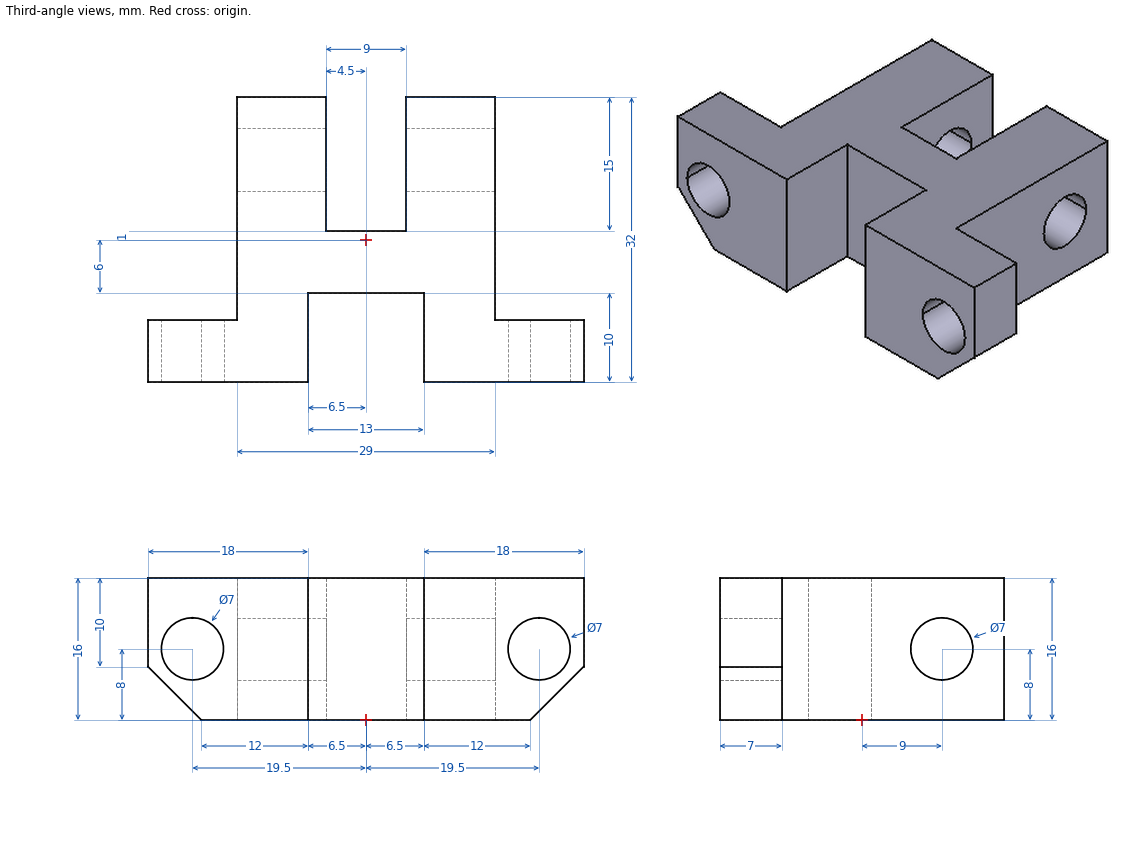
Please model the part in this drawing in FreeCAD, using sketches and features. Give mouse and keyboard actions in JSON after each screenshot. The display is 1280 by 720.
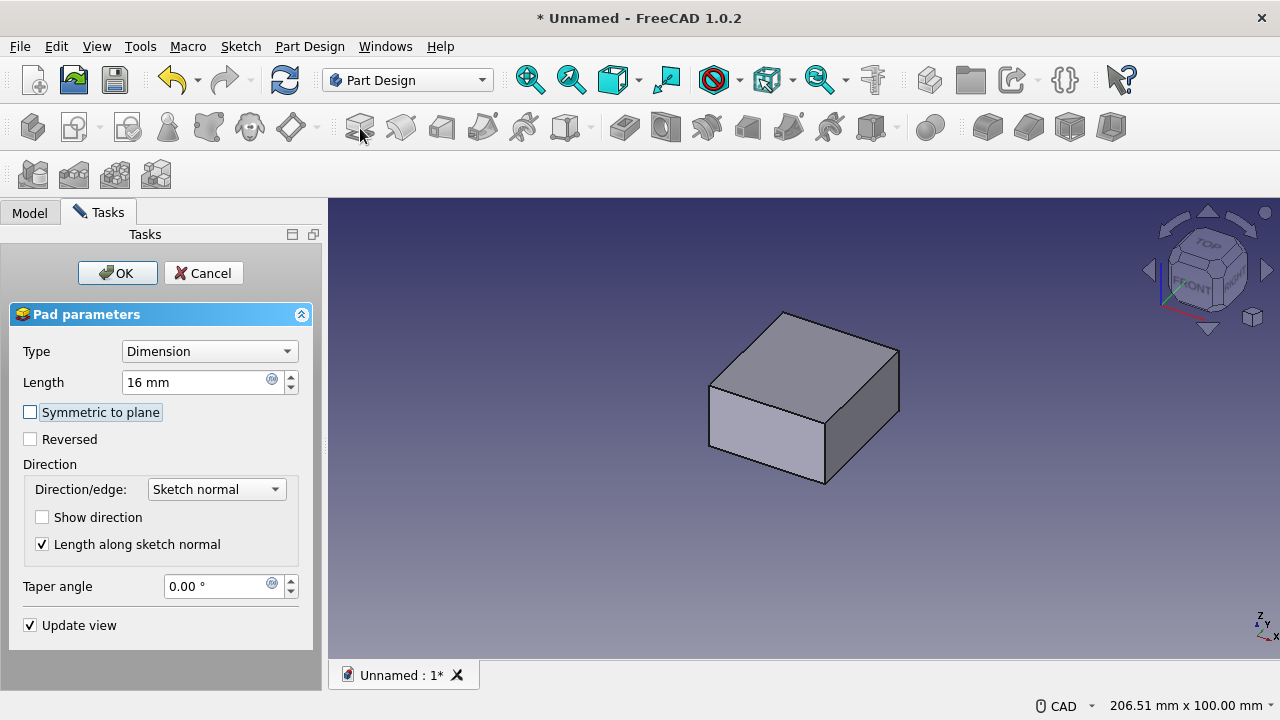
{"action": "left_click", "coordinate": [118, 273]}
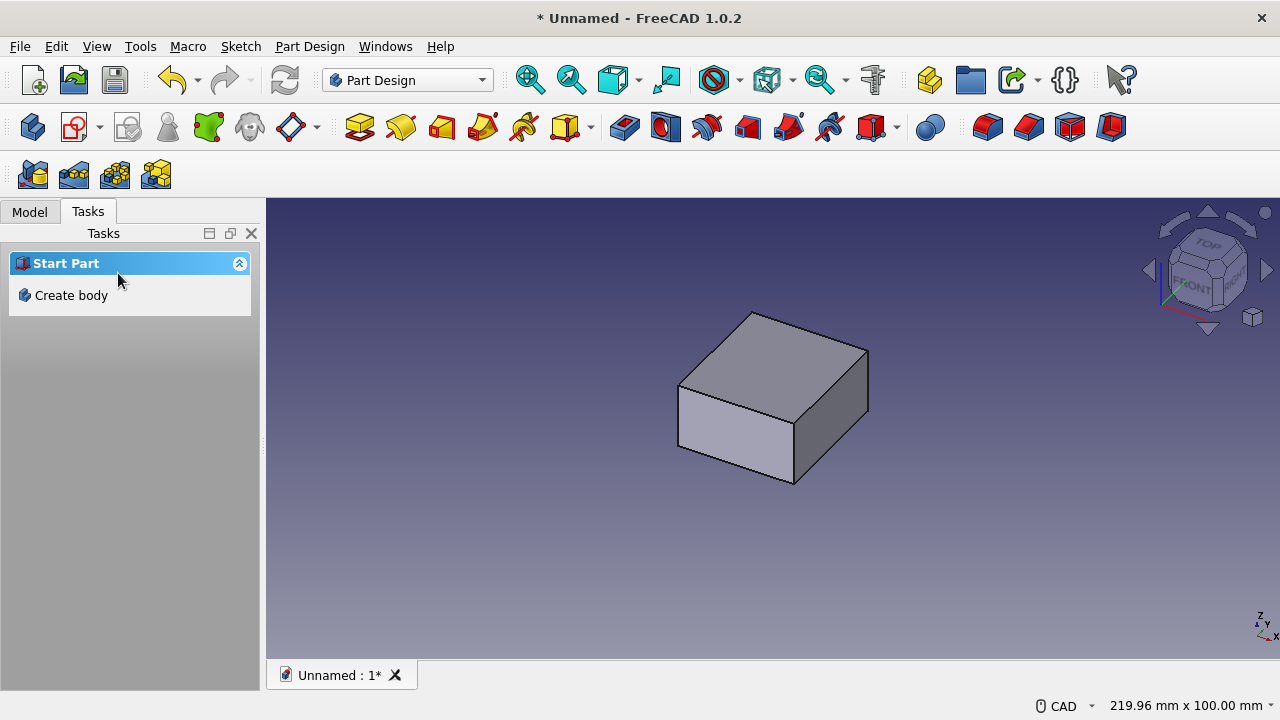
{"action": "left_click", "coordinate": [531, 80]}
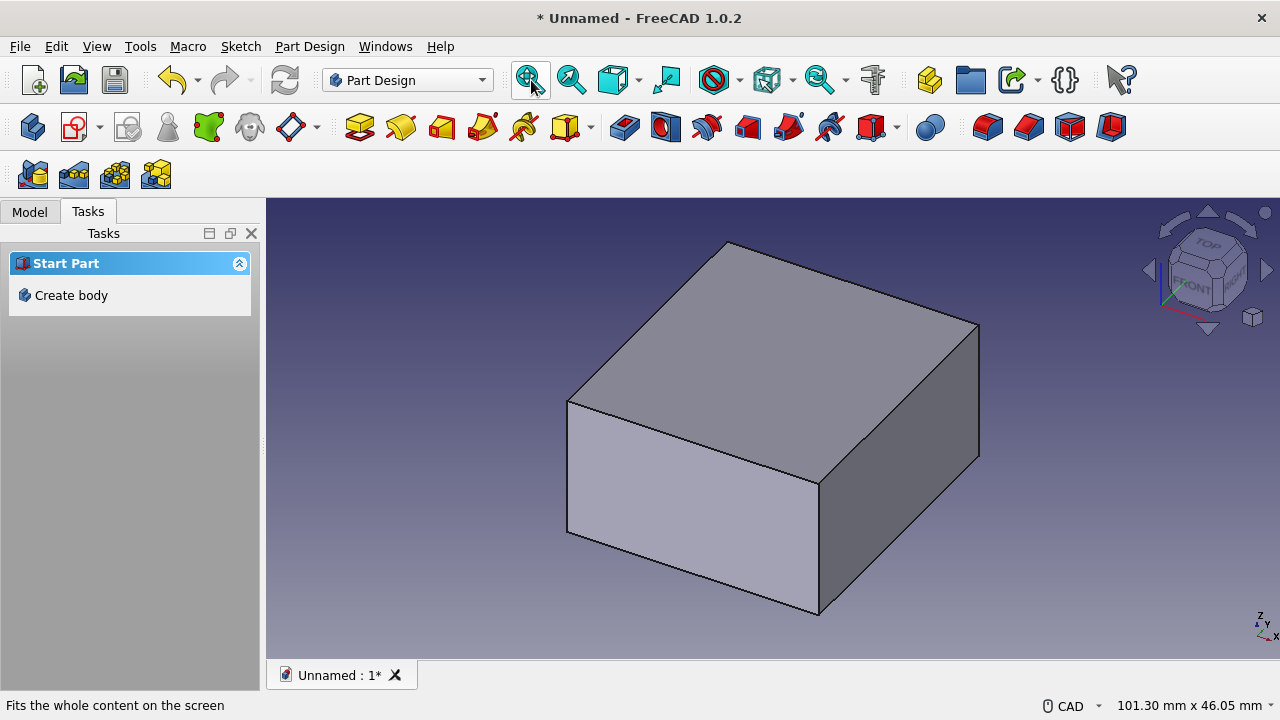
{"action": "left_click", "coordinate": [773, 362]}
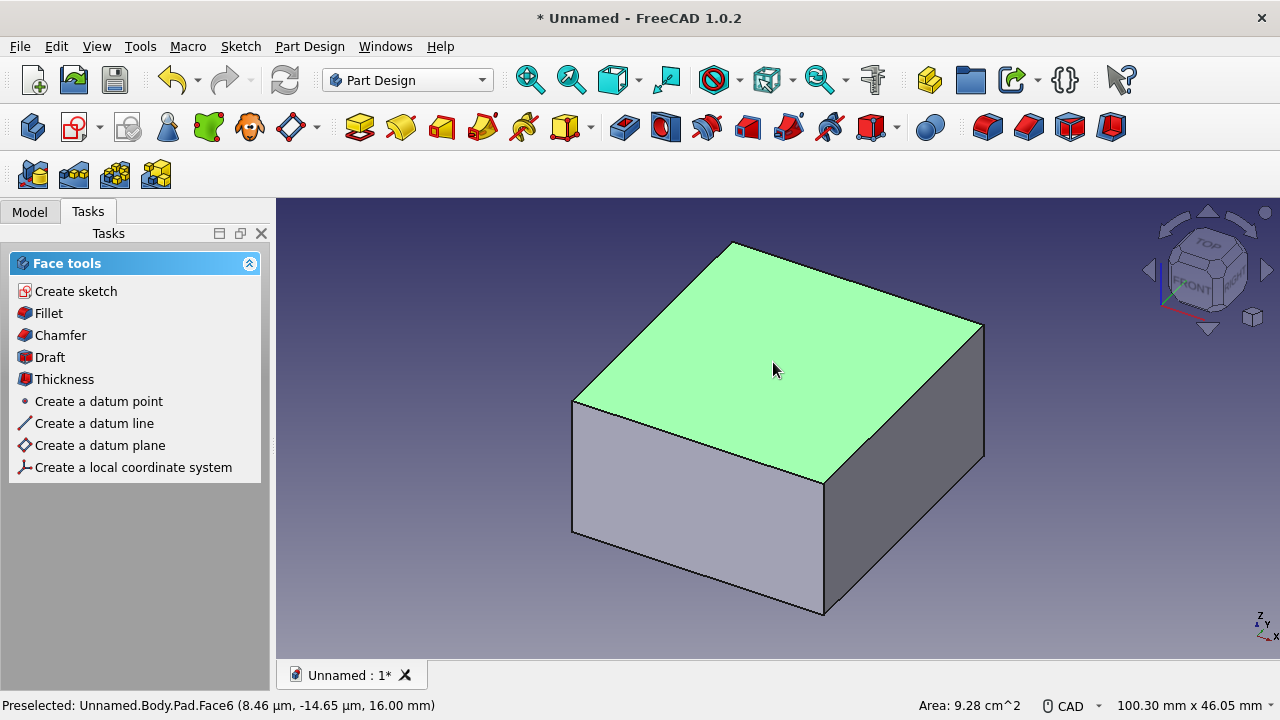
{"action": "left_click", "coordinate": [74, 128]}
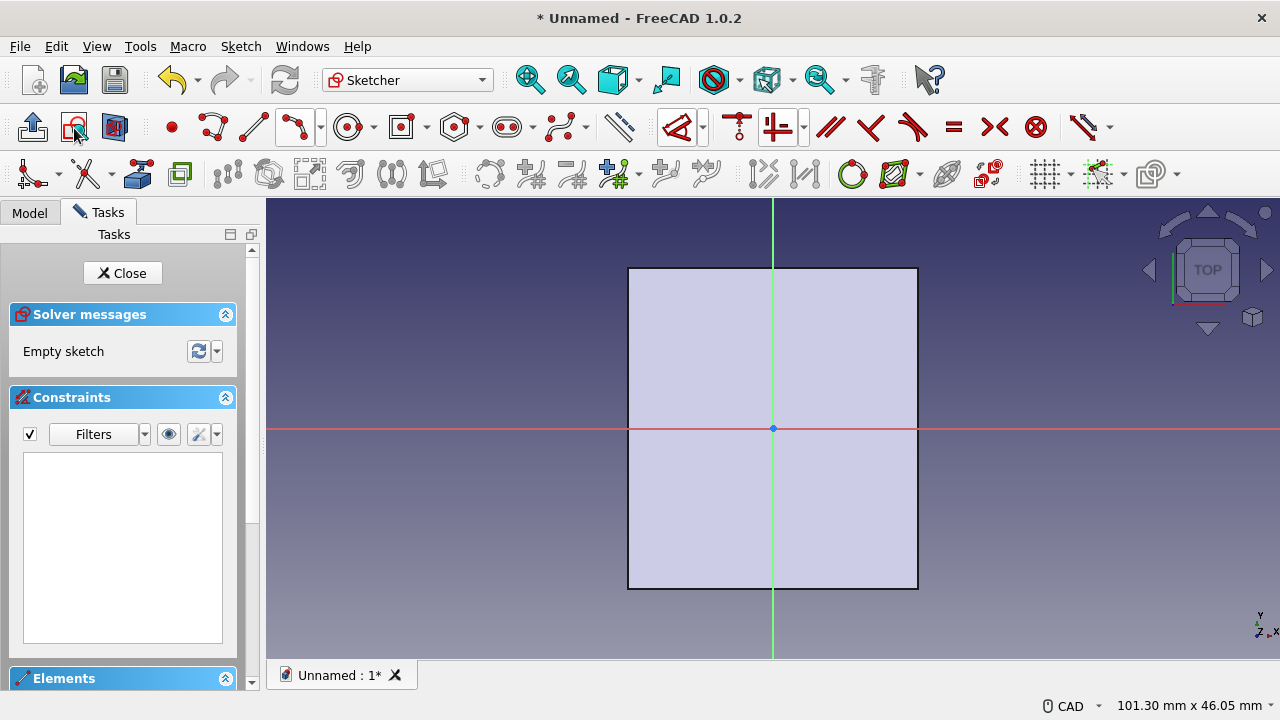
{"action": "scroll", "coordinate": [856, 606], "scroll_direction": "up", "scroll_amount": 3}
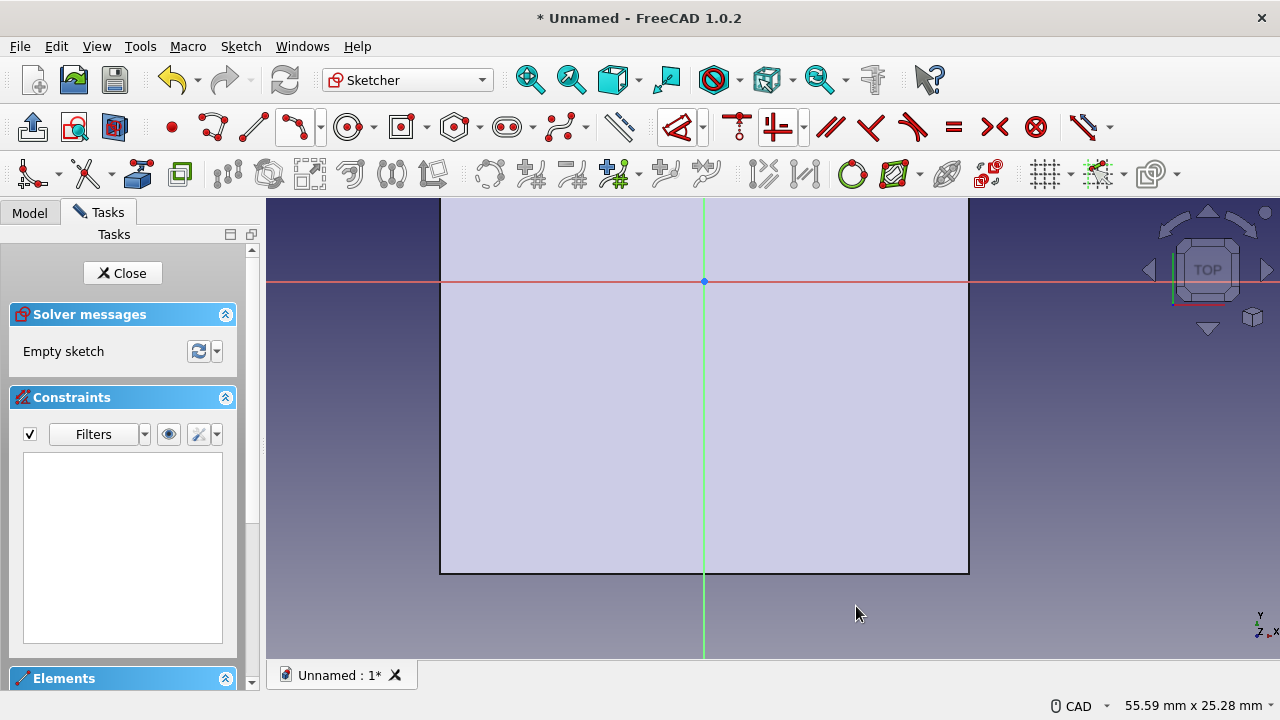
{"action": "left_click", "coordinate": [426, 128]}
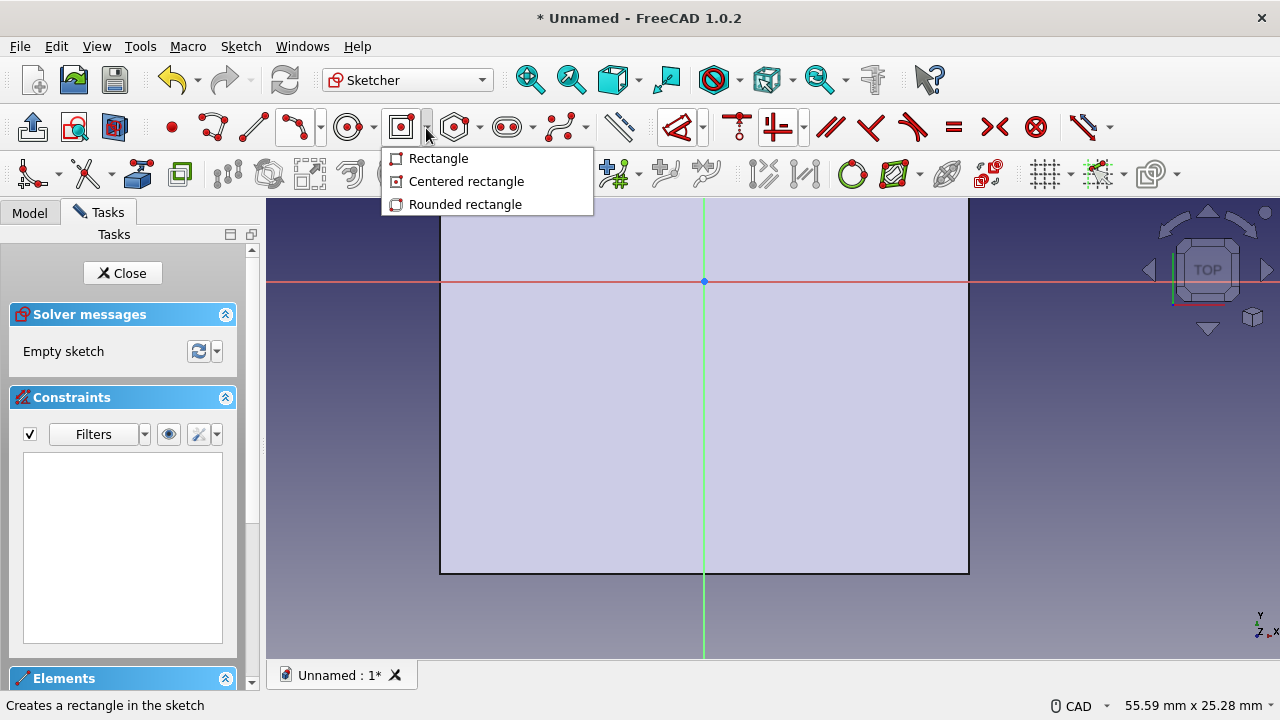
{"action": "left_click", "coordinate": [488, 158]}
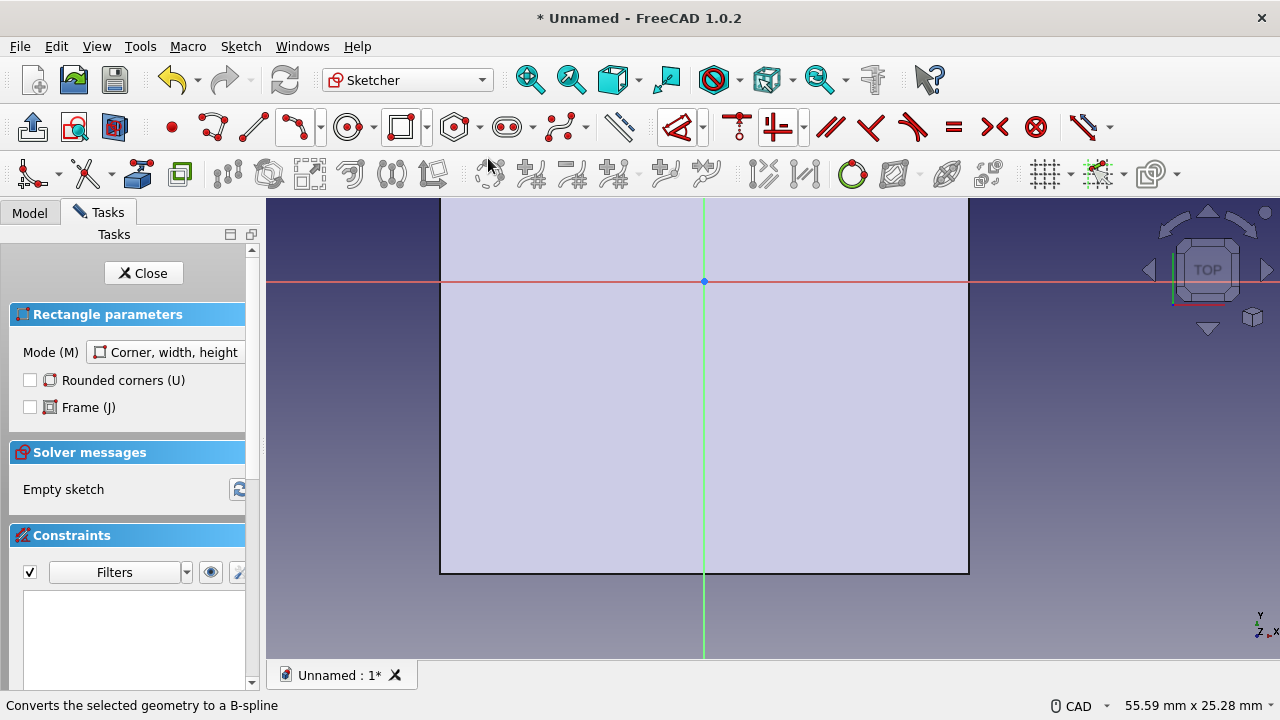
{"action": "left_click", "coordinate": [586, 391]}
{"action": "mouse_move", "coordinate": [823, 574]}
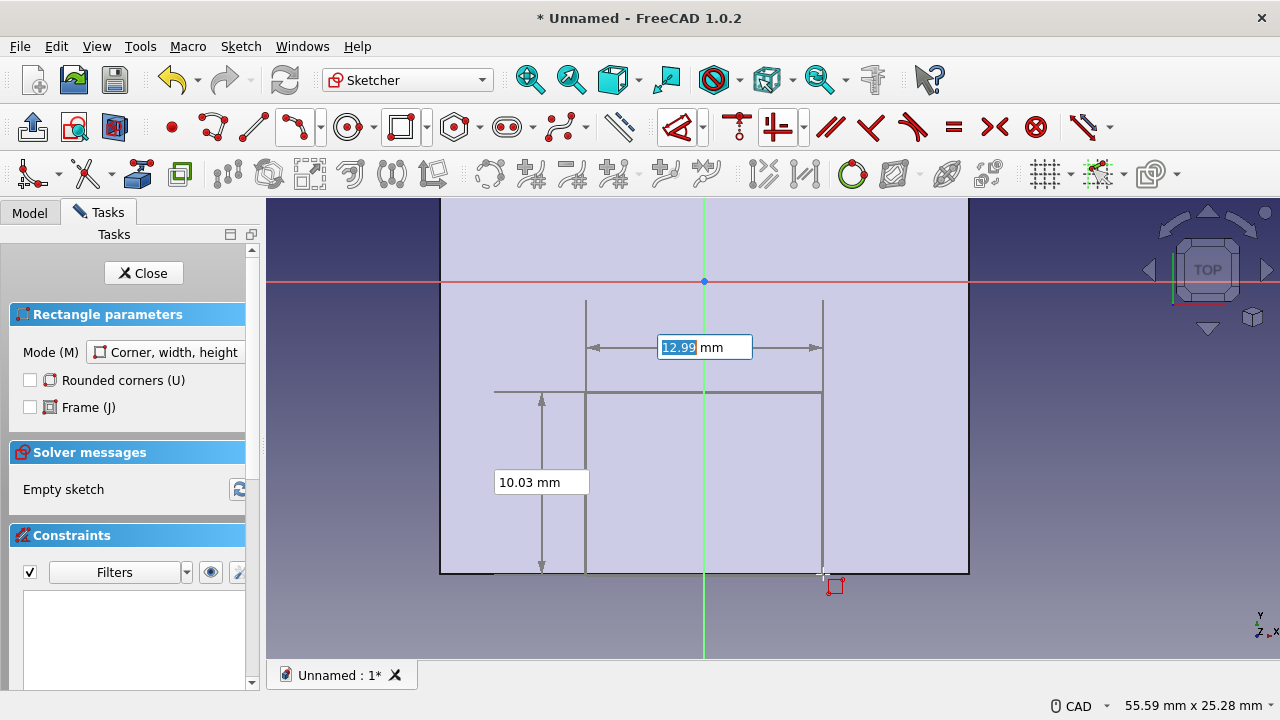
{"action": "type", "text": "13"}
{"action": "key", "text": "Tab"}
{"action": "type", "text": "10"}
{"action": "key", "text": "Return"}
{"action": "key", "text": "Escape"}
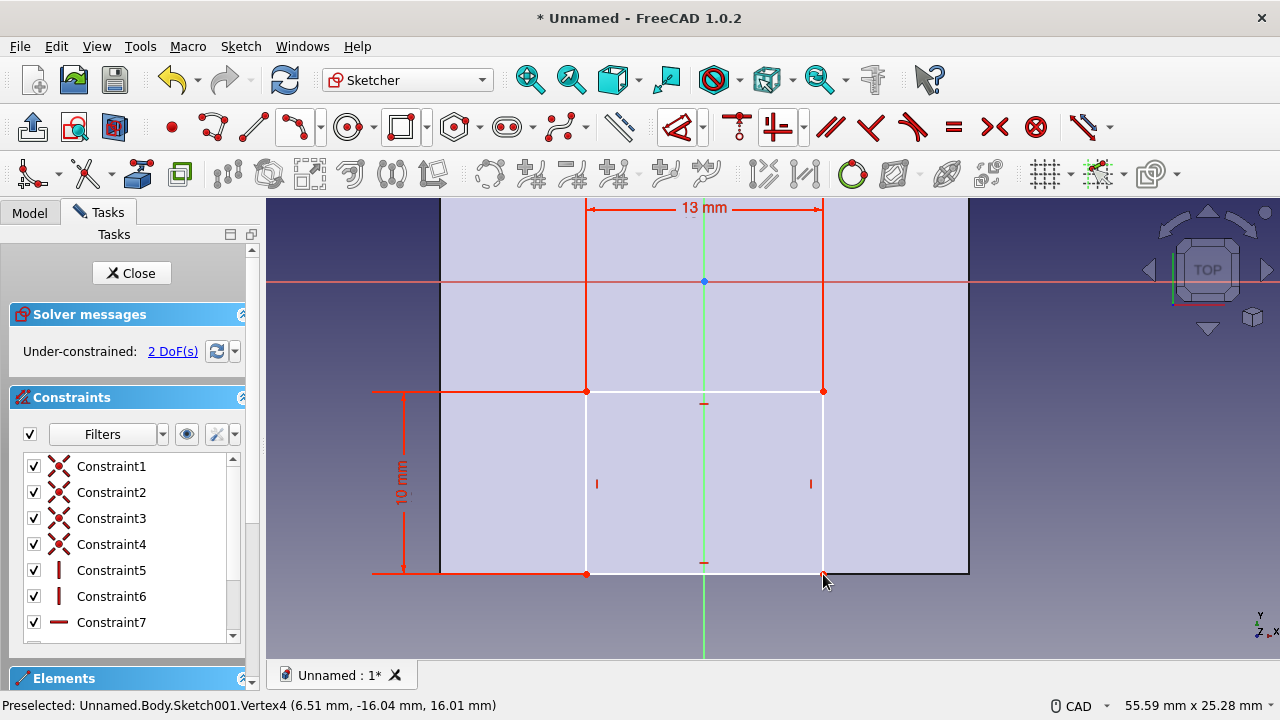
{"action": "left_click", "coordinate": [676, 128]}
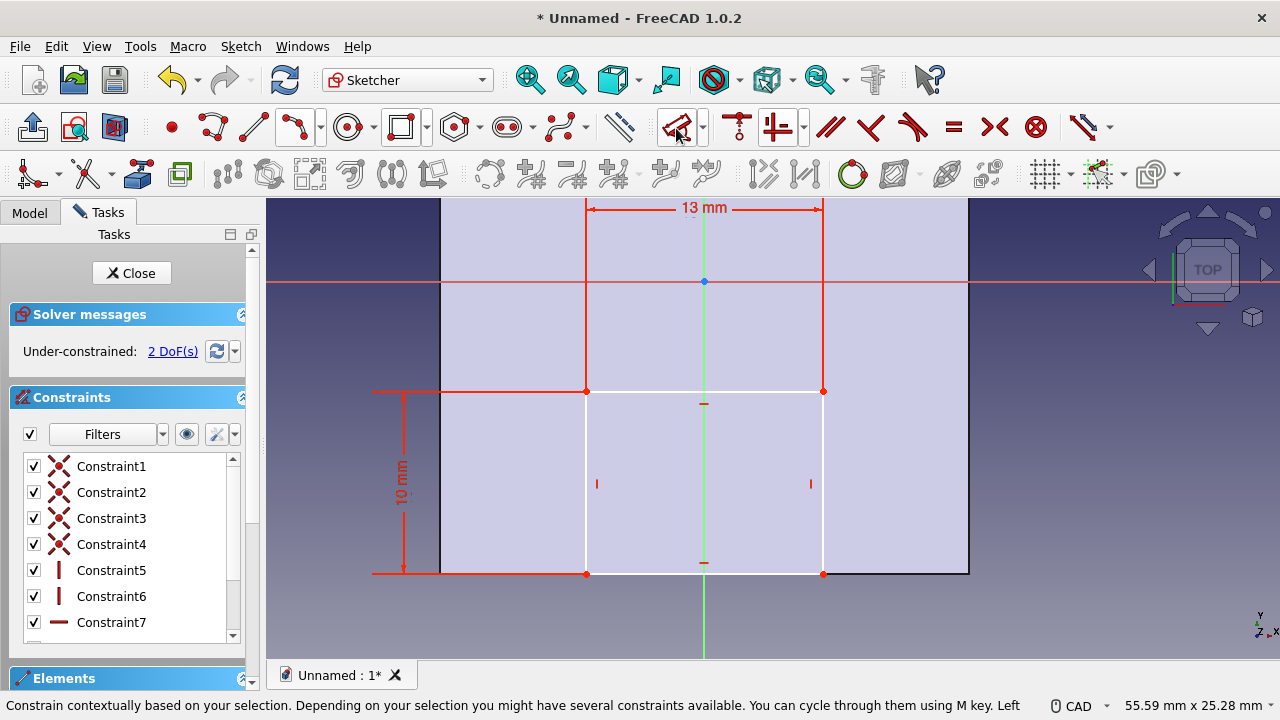
{"action": "left_click", "coordinate": [586, 392]}
{"action": "left_click", "coordinate": [552, 337]}